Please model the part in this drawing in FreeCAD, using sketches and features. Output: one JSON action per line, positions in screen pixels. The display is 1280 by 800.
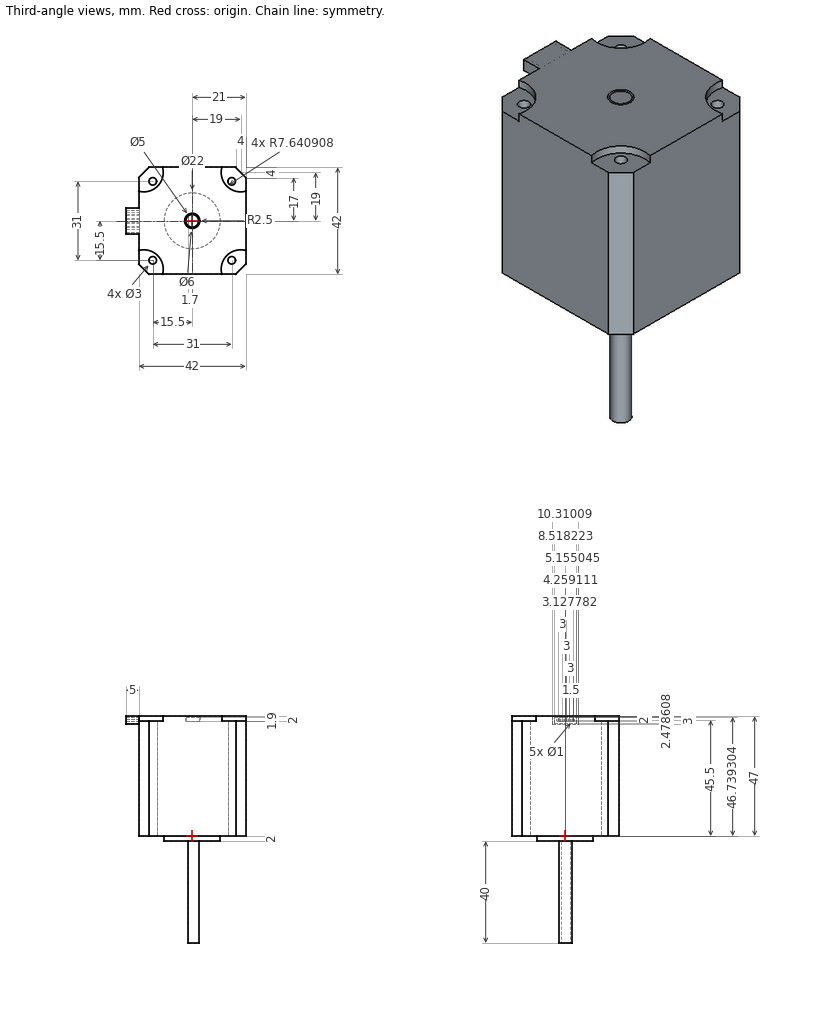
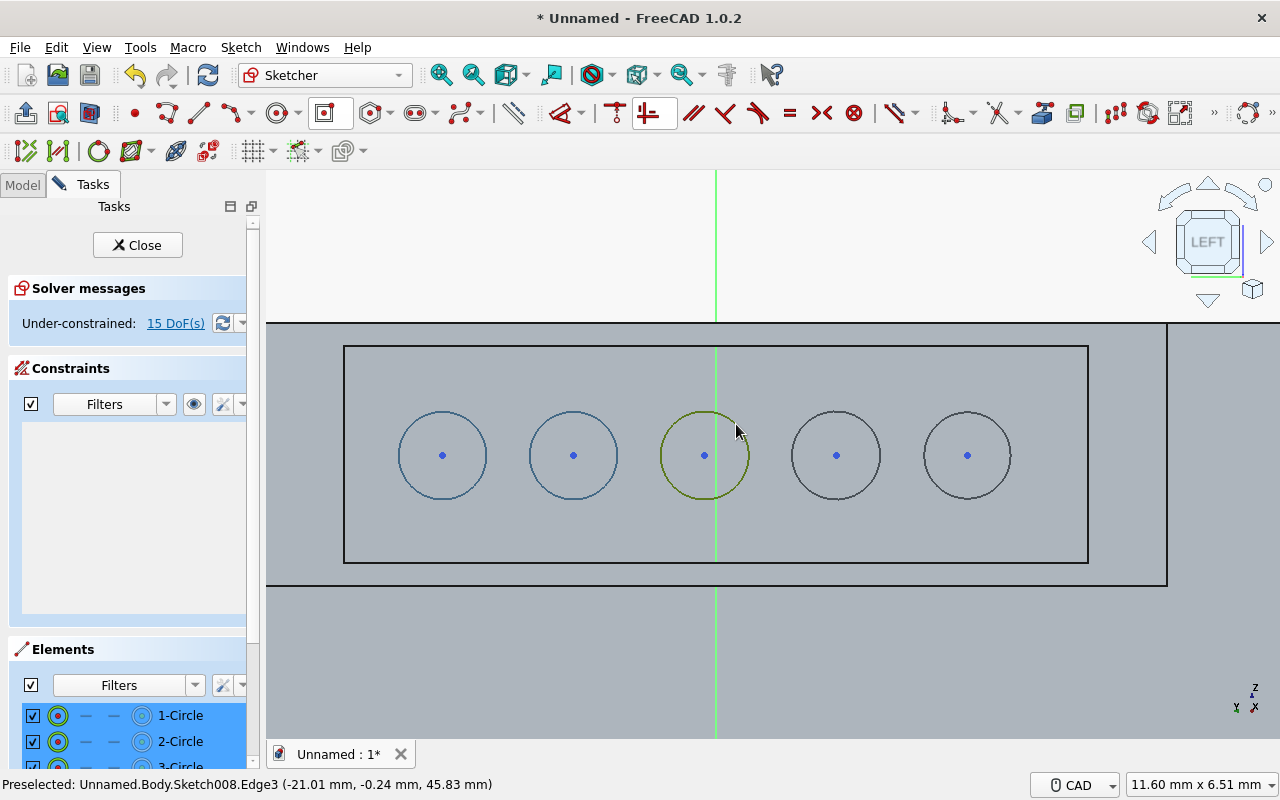
{"action": "left_click", "coordinate": [867, 424]}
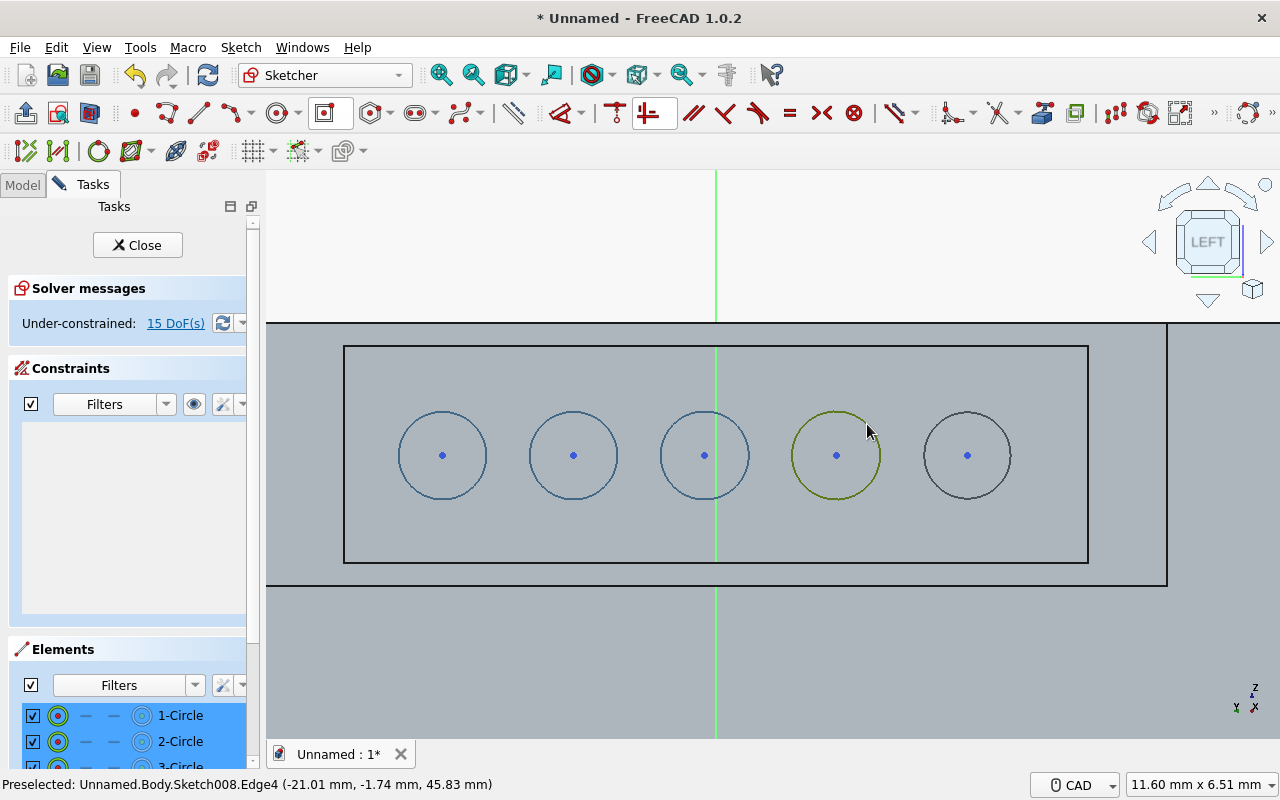
{"action": "left_click", "coordinate": [998, 425]}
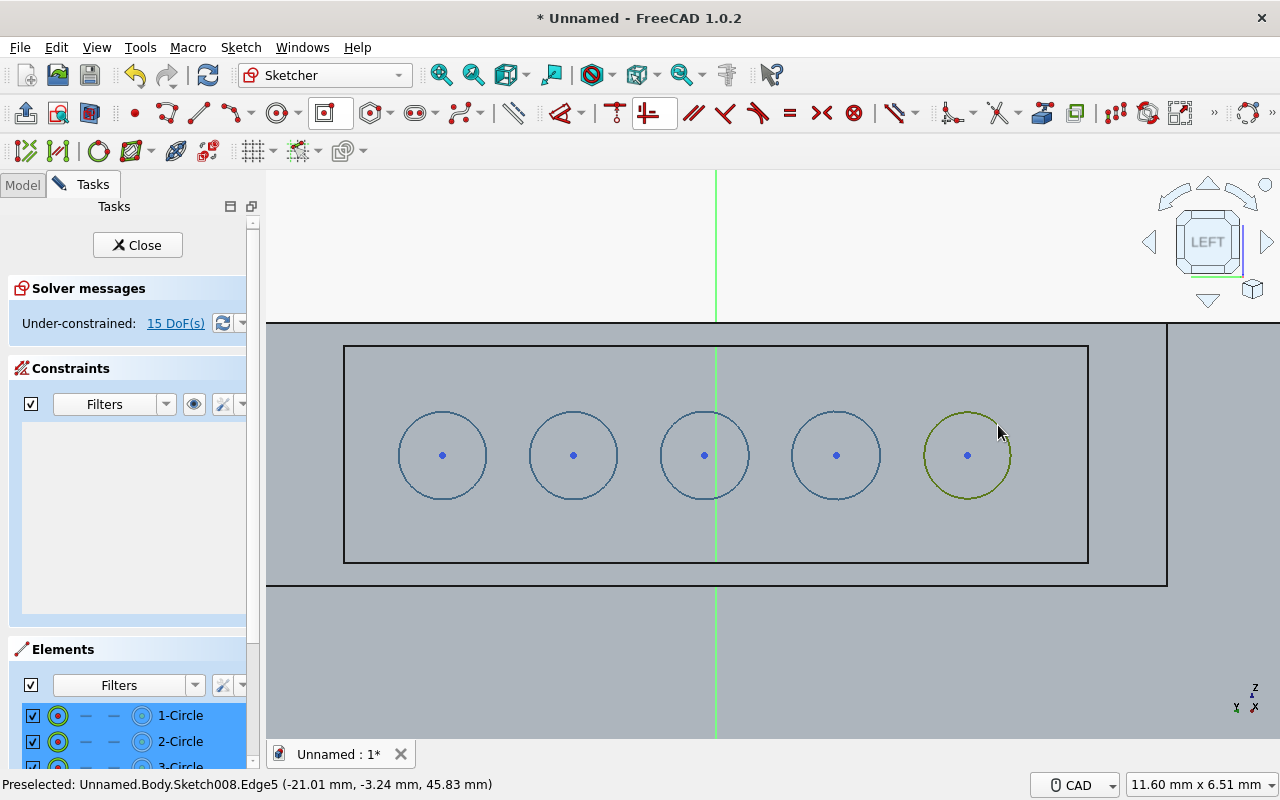
{"action": "left_click", "coordinate": [790, 114]}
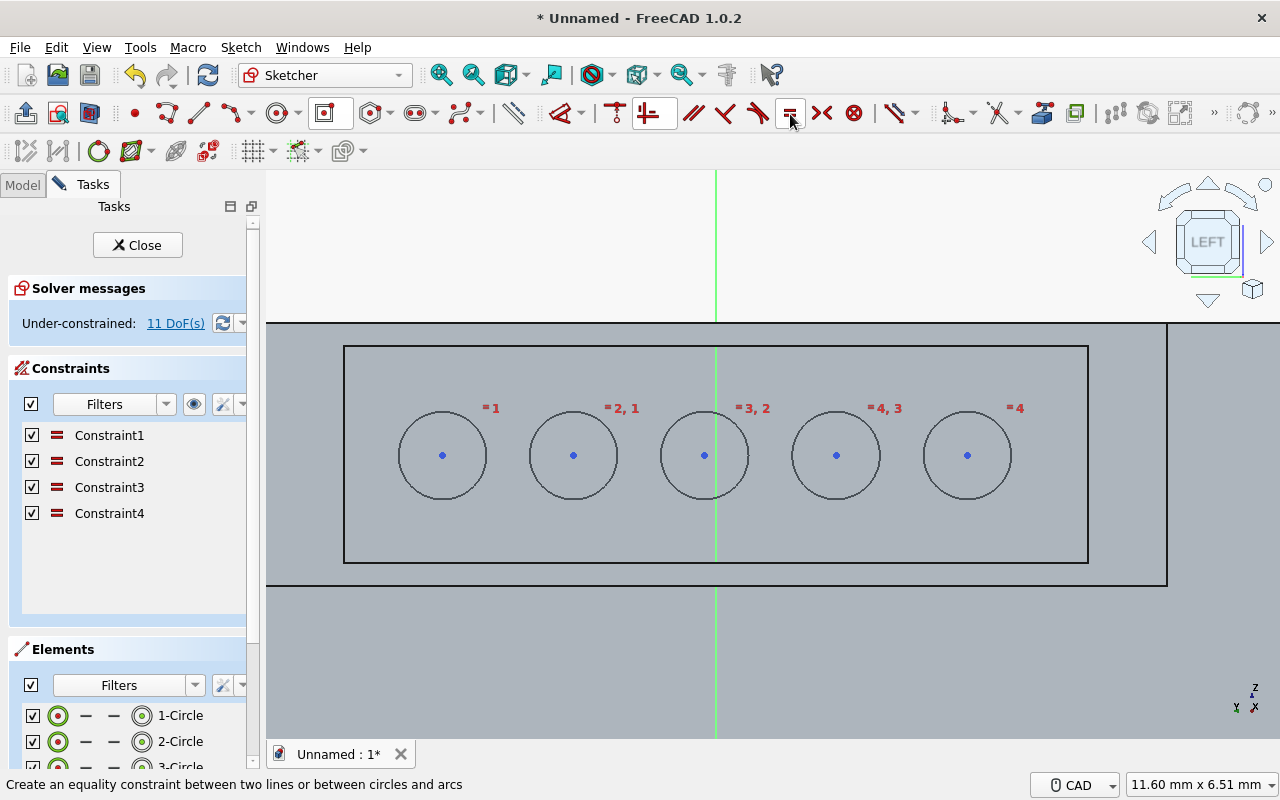
{"action": "left_click", "coordinate": [443, 456]}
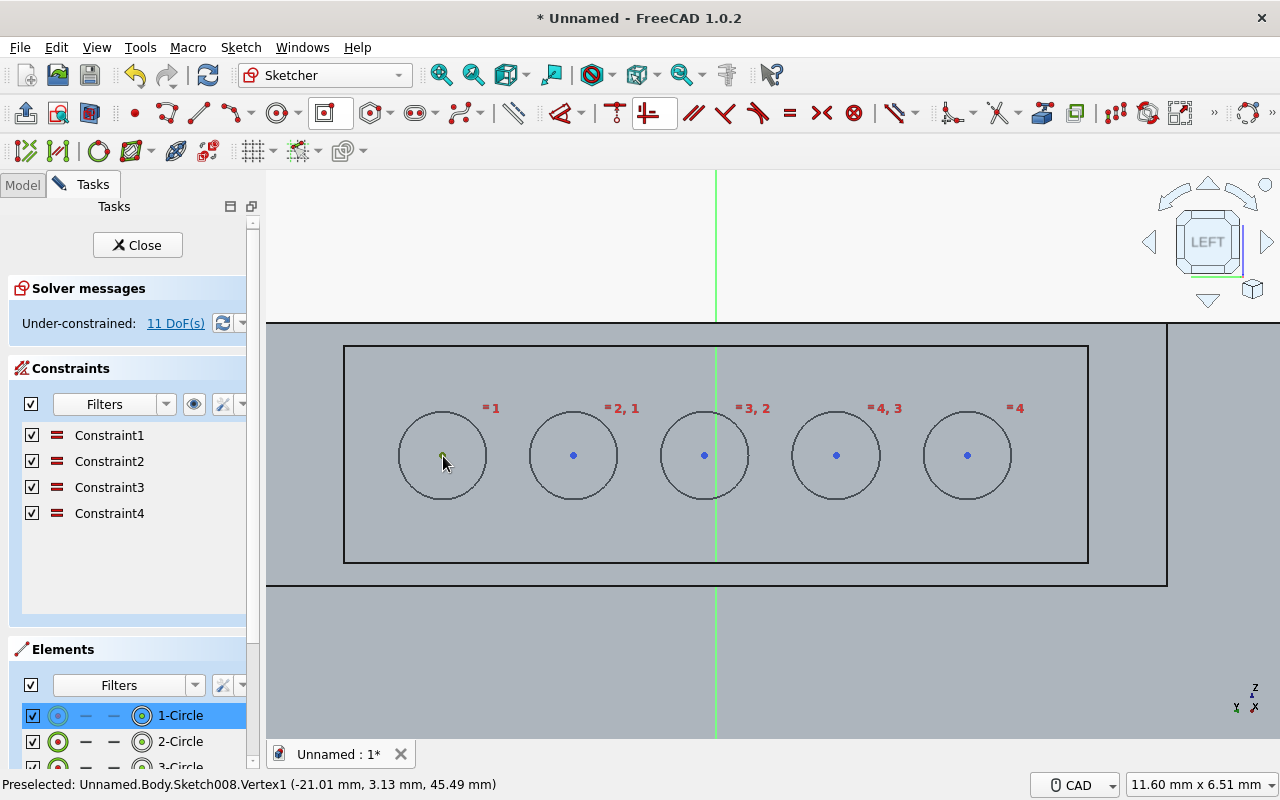
{"action": "left_click", "coordinate": [574, 456]}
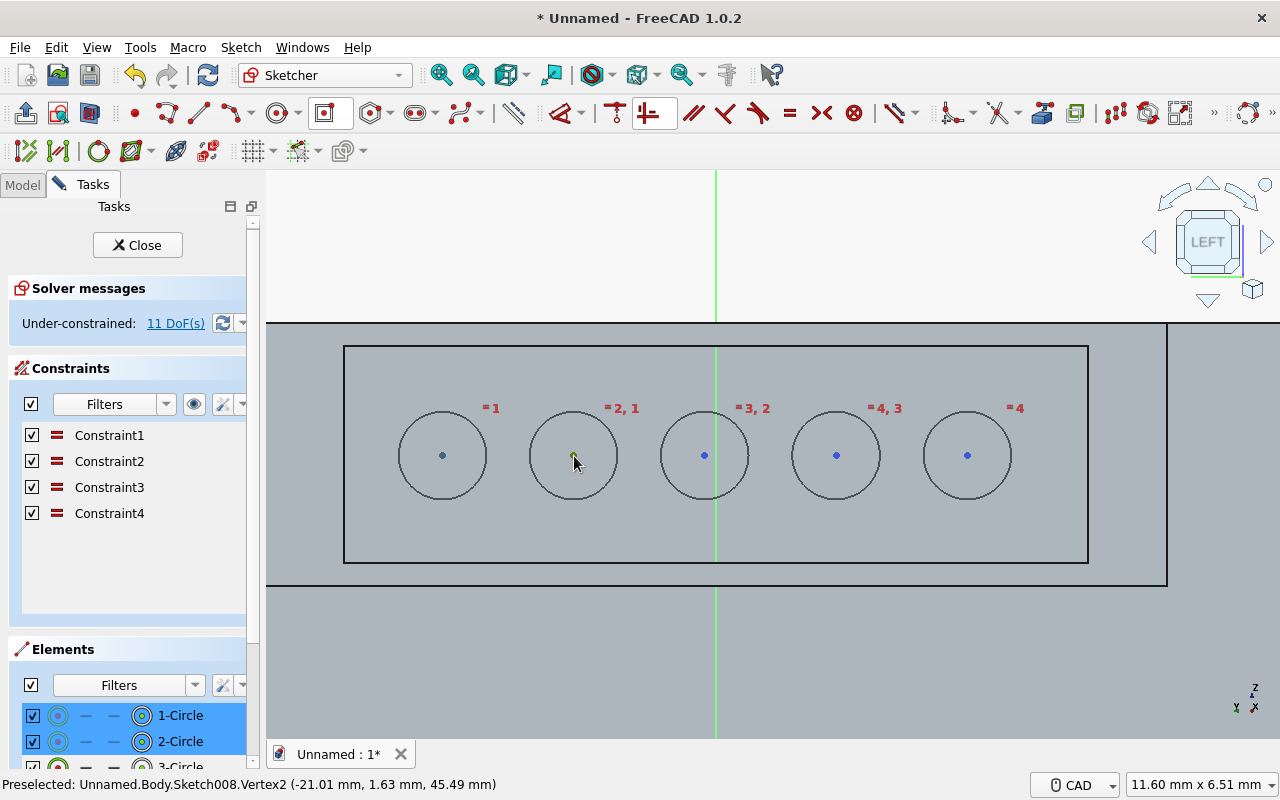
{"action": "key", "text": "h"}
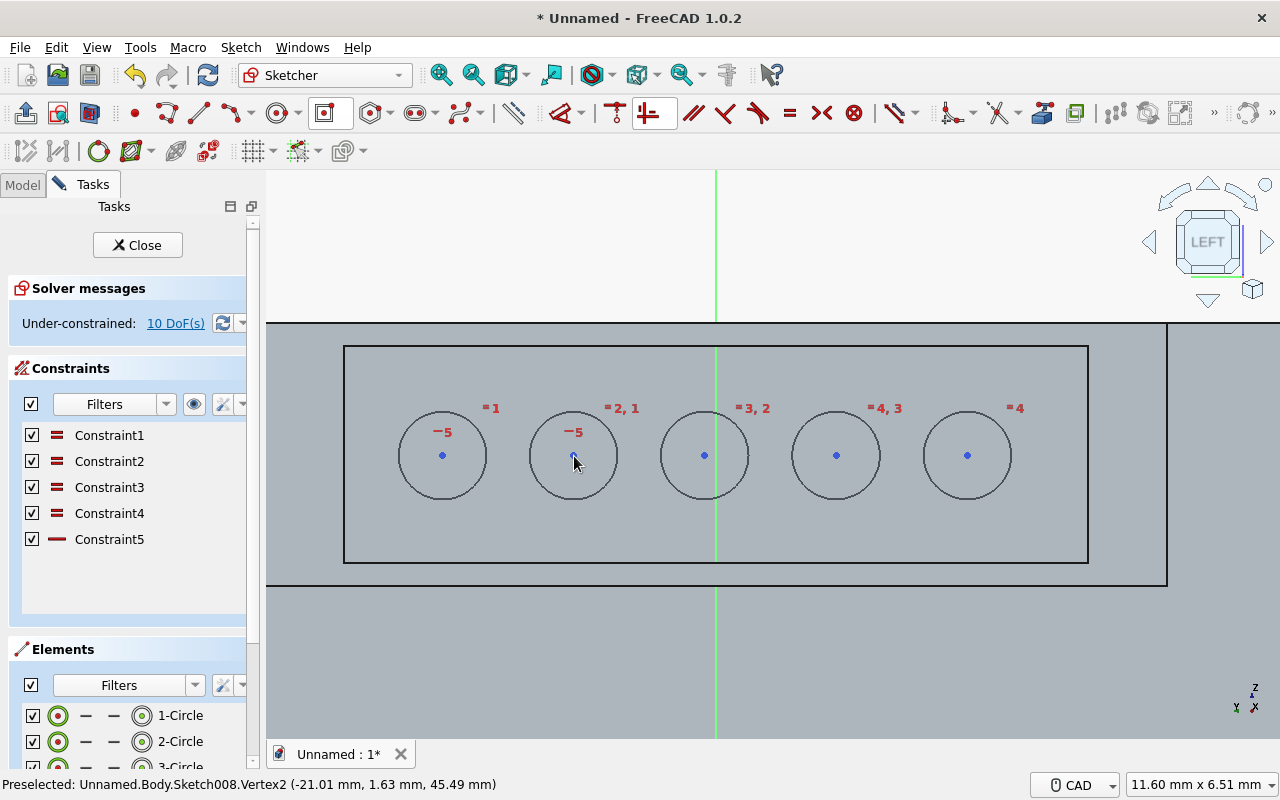
{"action": "left_click", "coordinate": [574, 456]}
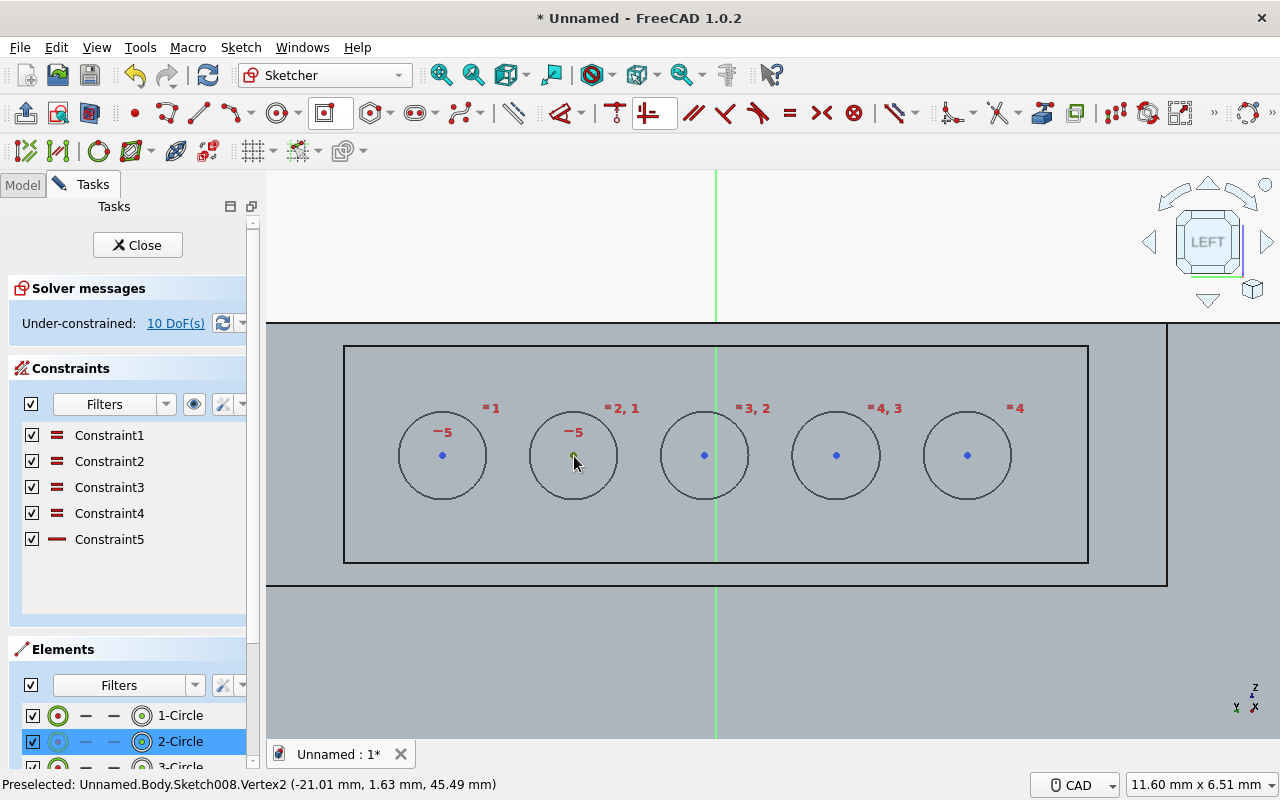
{"action": "left_click", "coordinate": [705, 455]}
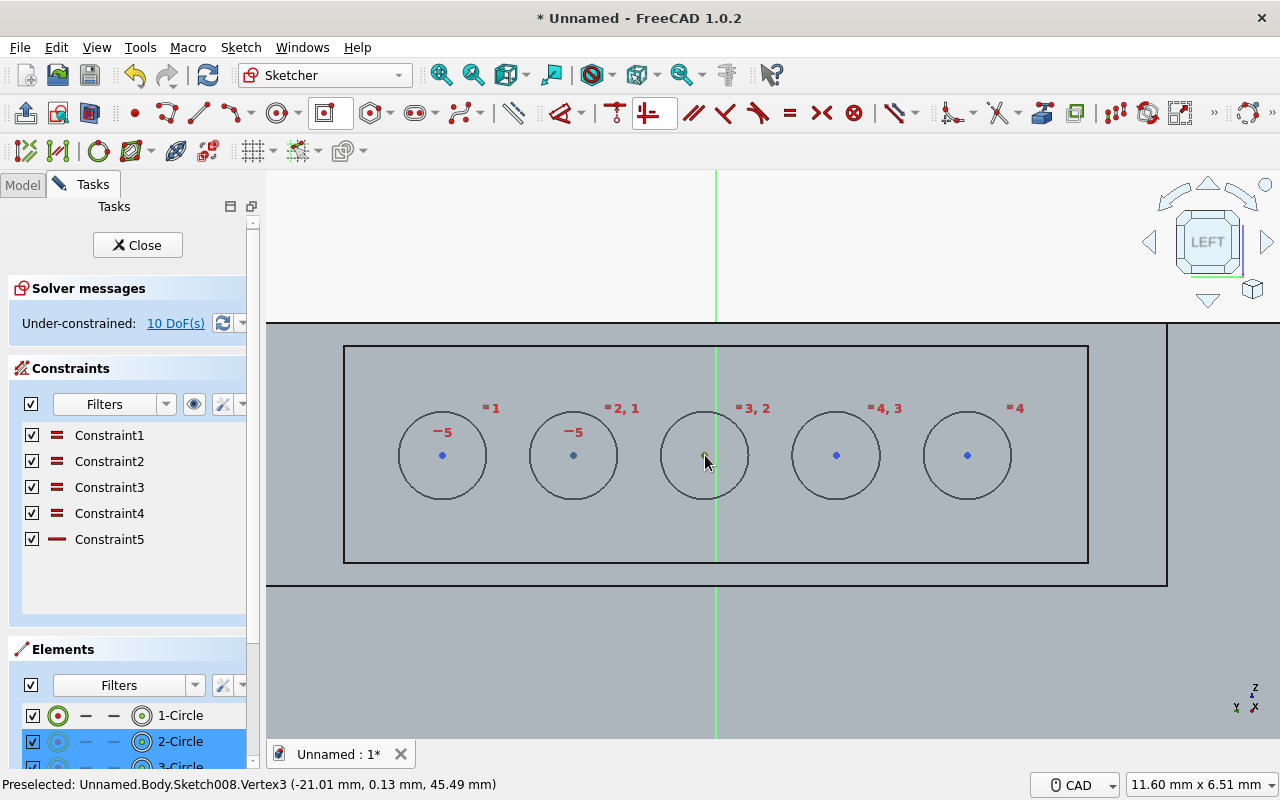
{"action": "left_click", "coordinate": [672, 114]}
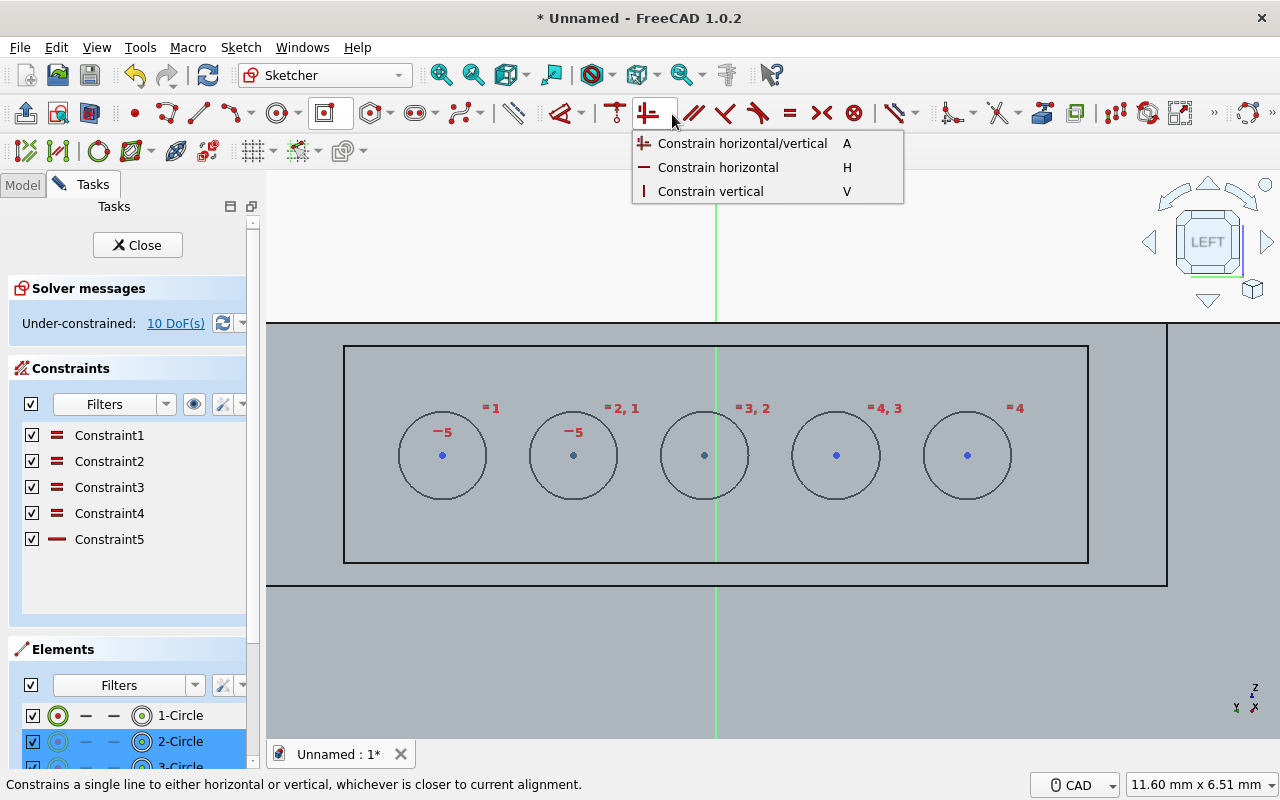
{"action": "left_click", "coordinate": [768, 167]}